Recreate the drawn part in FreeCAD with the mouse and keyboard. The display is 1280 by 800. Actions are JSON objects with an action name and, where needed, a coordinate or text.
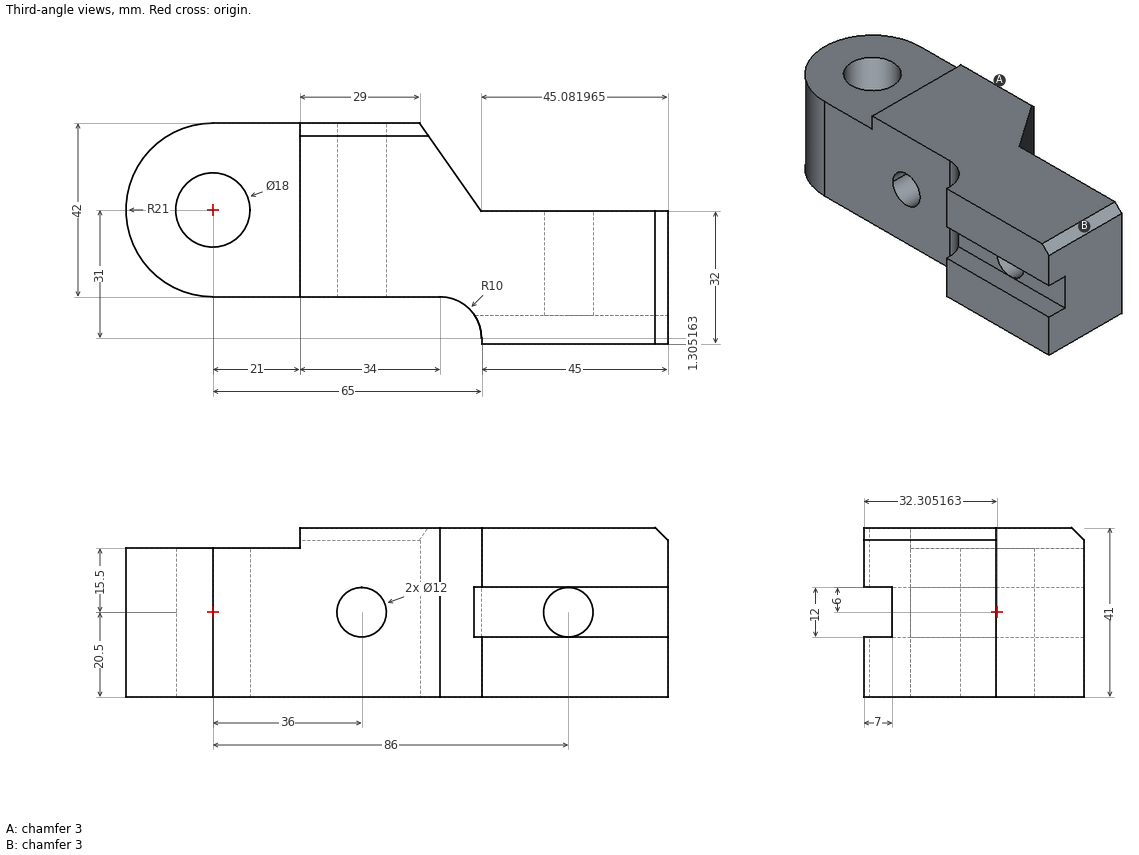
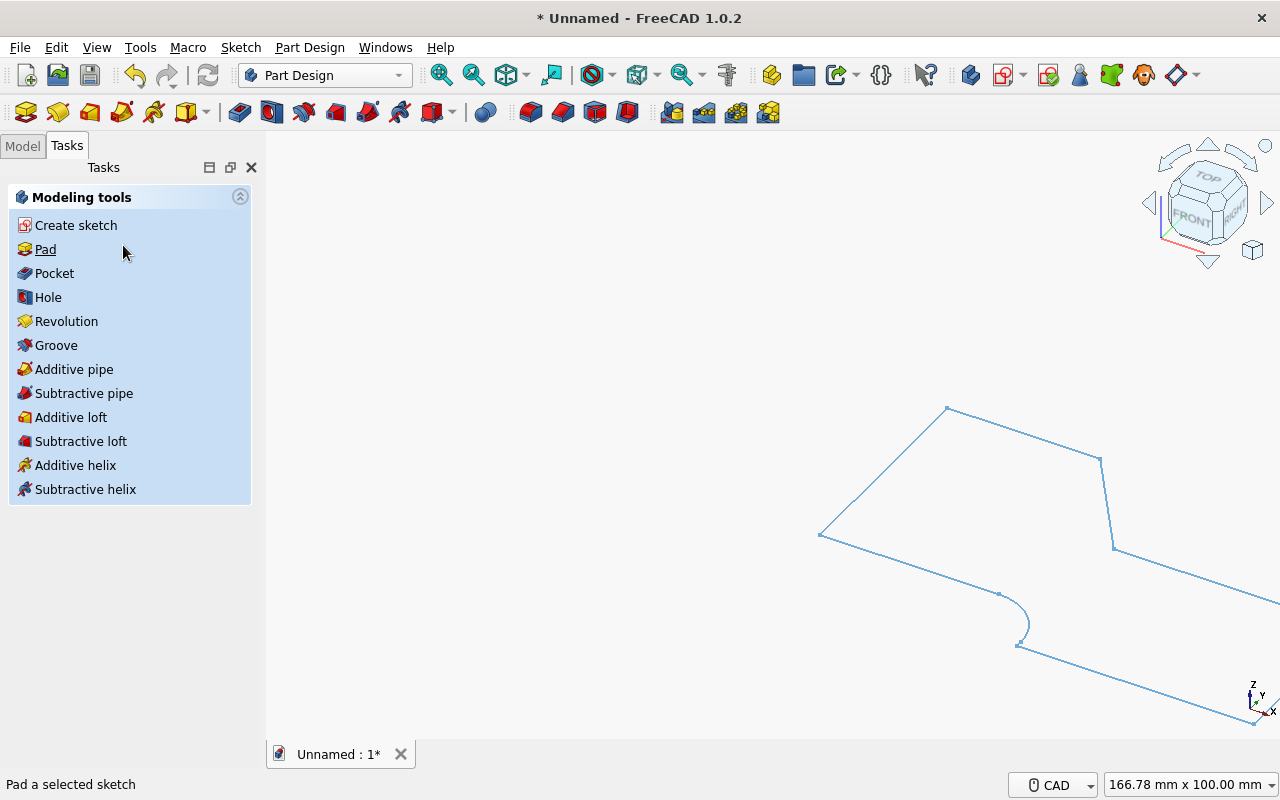
{"action": "left_click", "coordinate": [26, 112]}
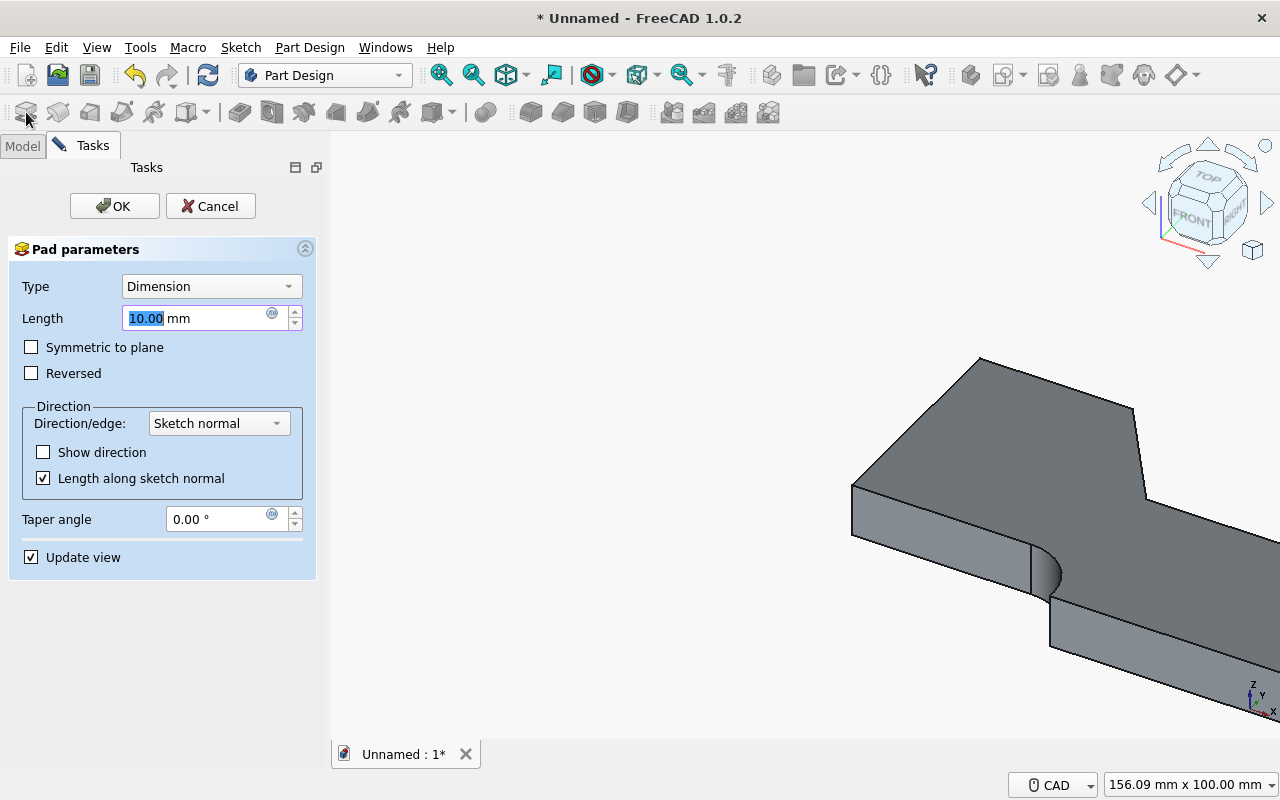
{"action": "type", "text": "41"}
{"action": "key", "text": "Tab"}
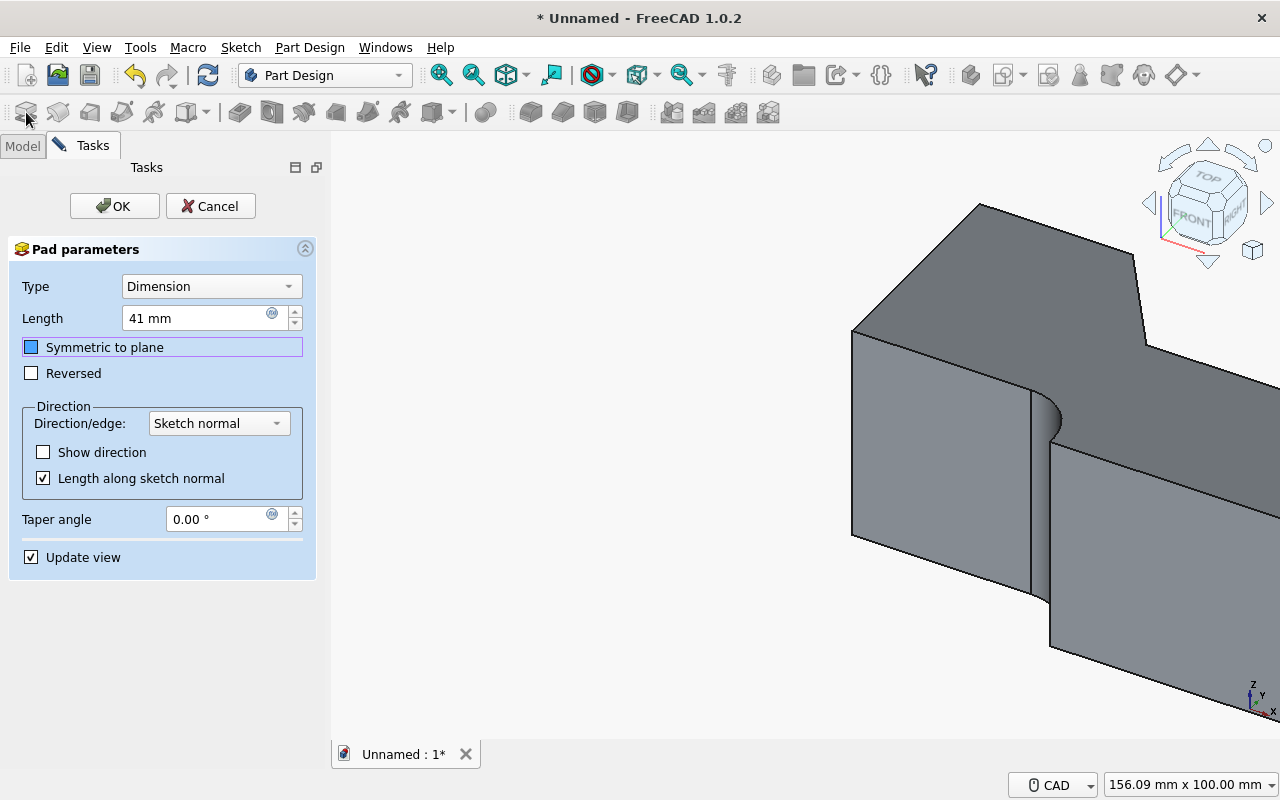
{"action": "left_click", "coordinate": [30, 347]}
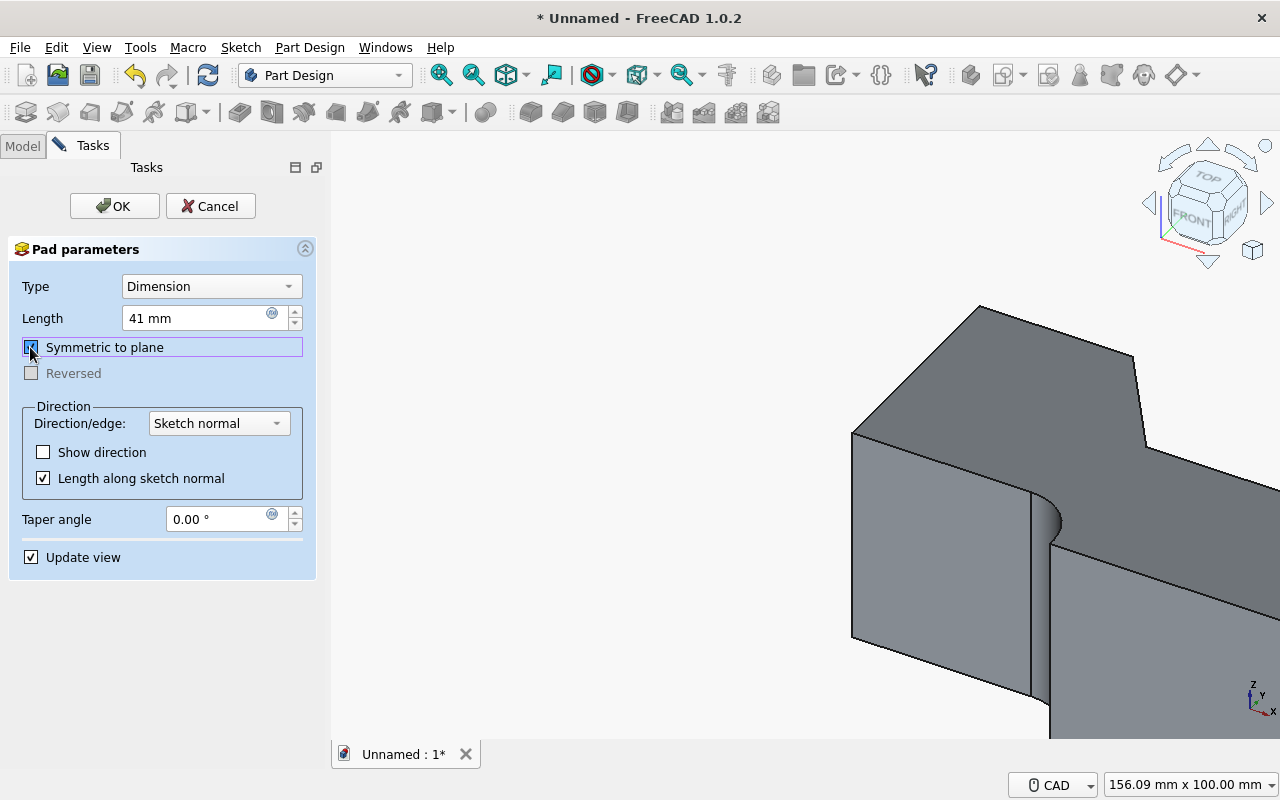
{"action": "left_click", "coordinate": [115, 206]}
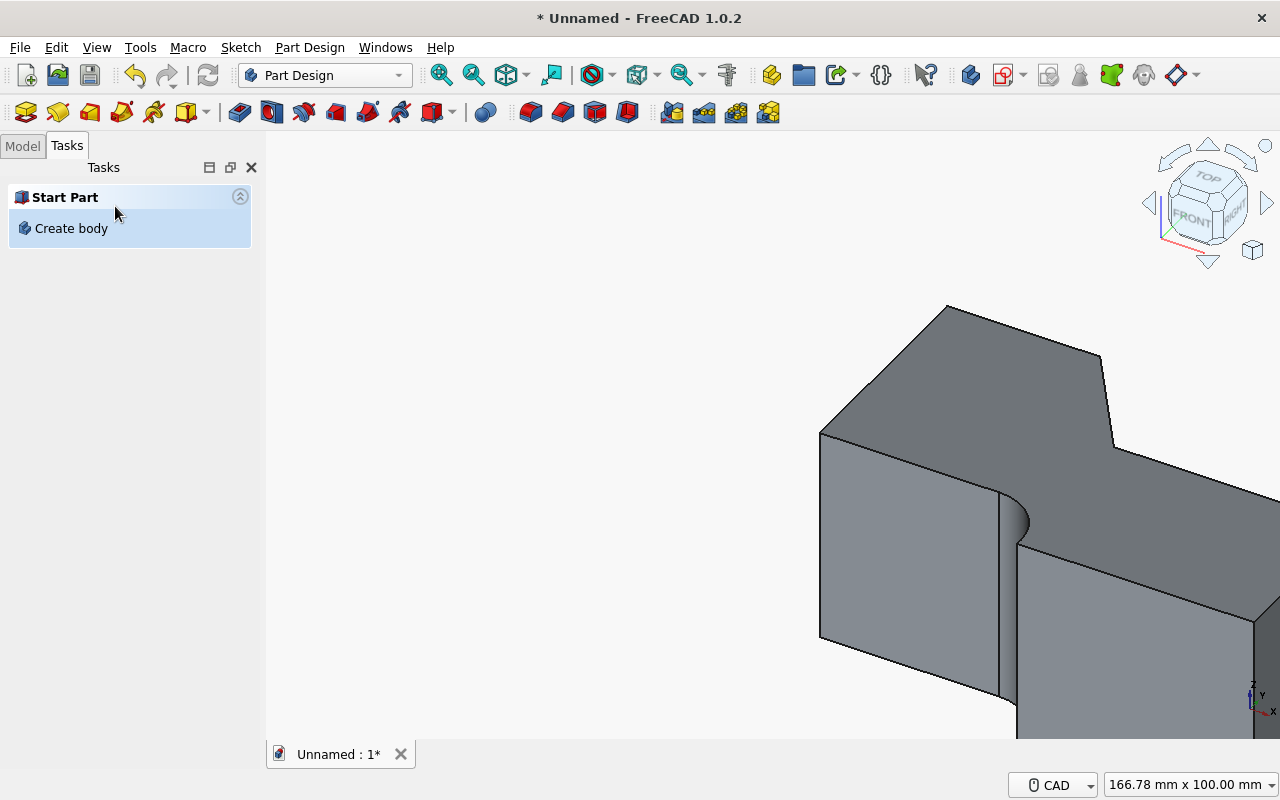
{"action": "left_click", "coordinate": [442, 76]}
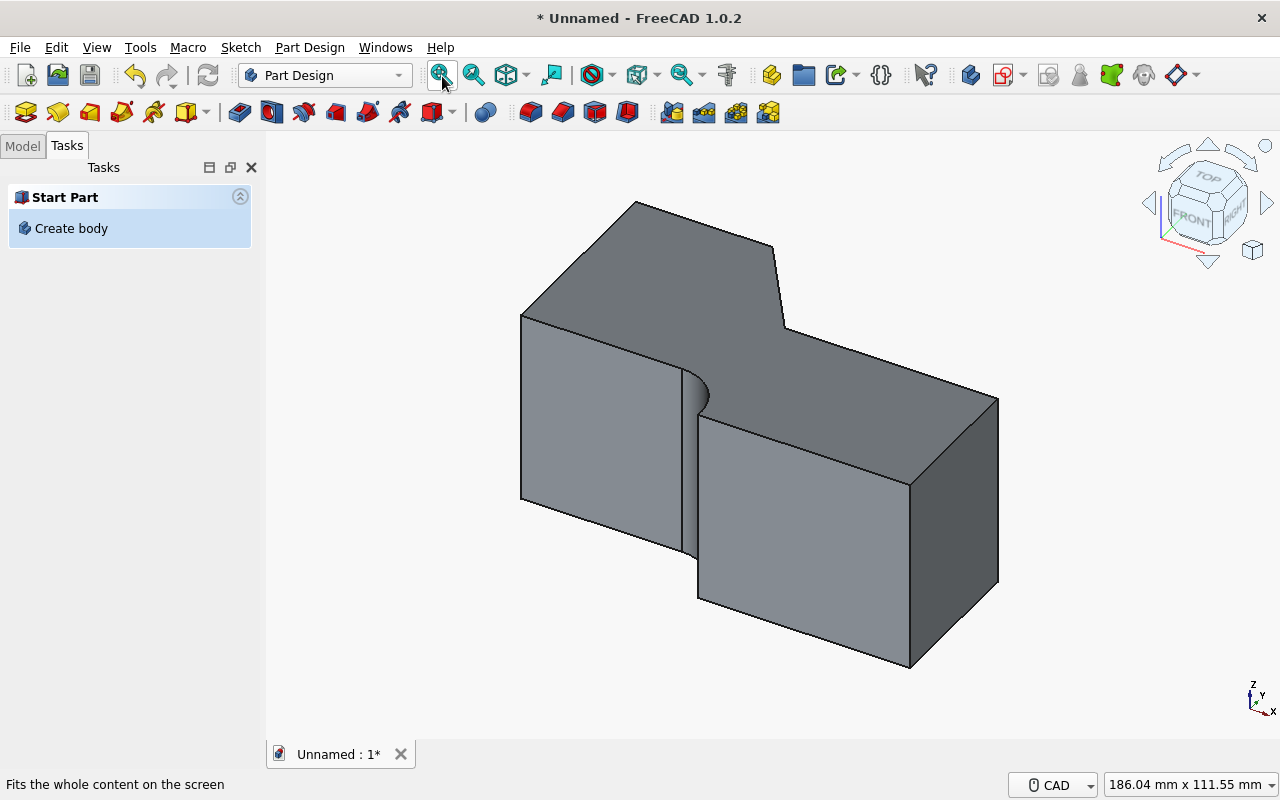
{"action": "left_click", "coordinate": [1004, 76]}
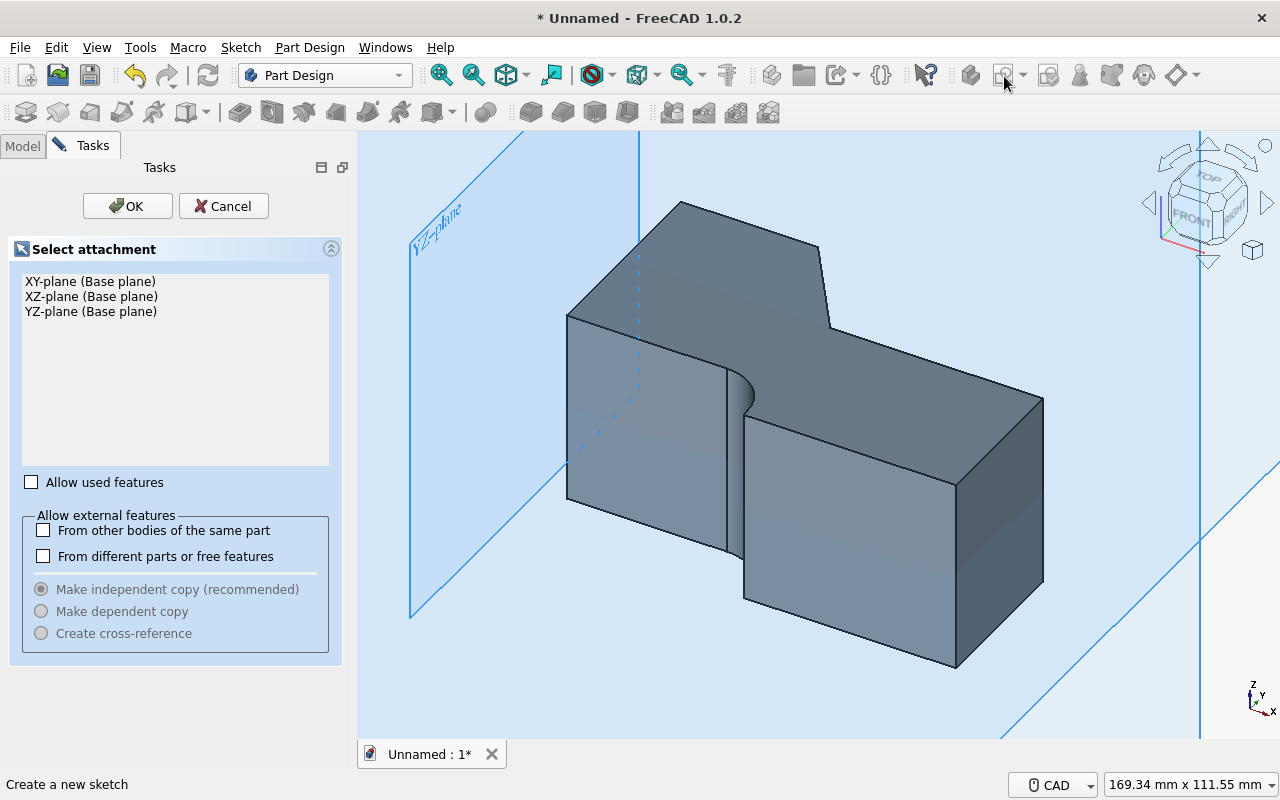
{"action": "left_click", "coordinate": [82, 282]}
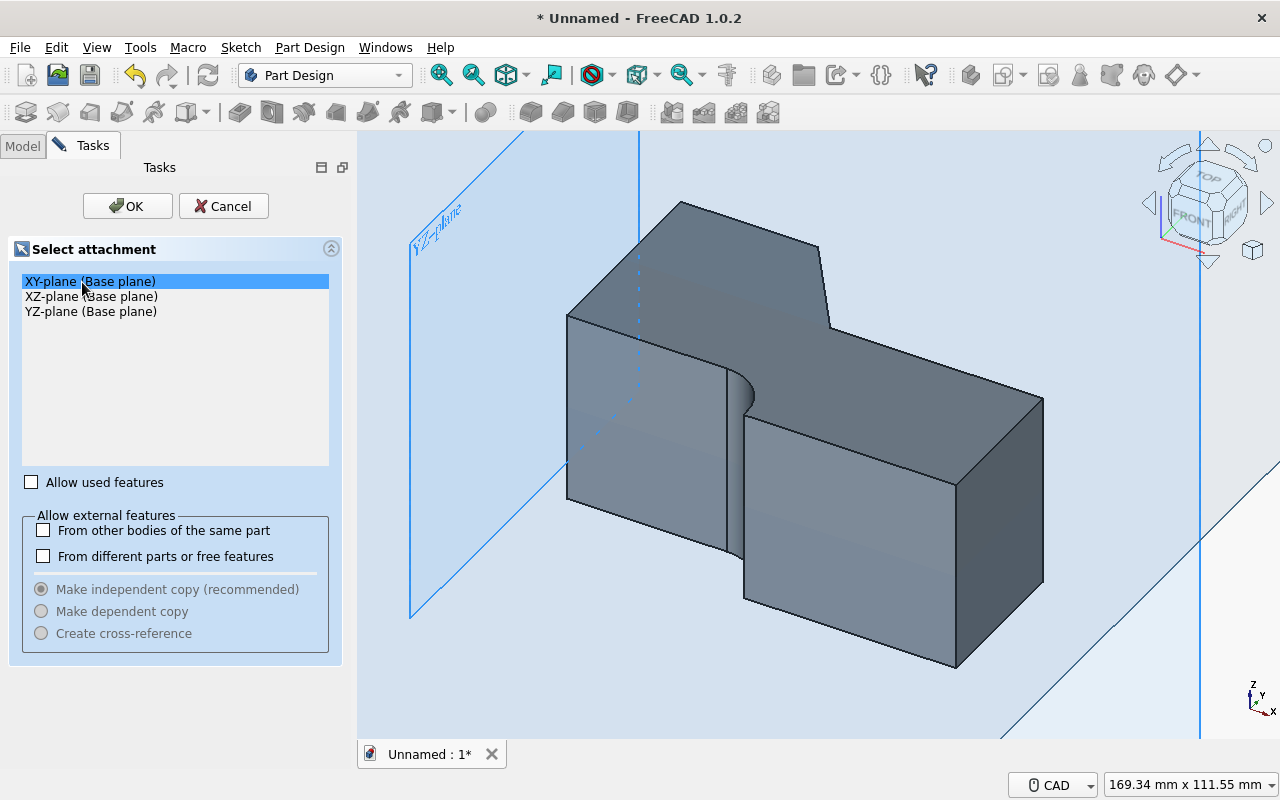
{"action": "left_click", "coordinate": [128, 206]}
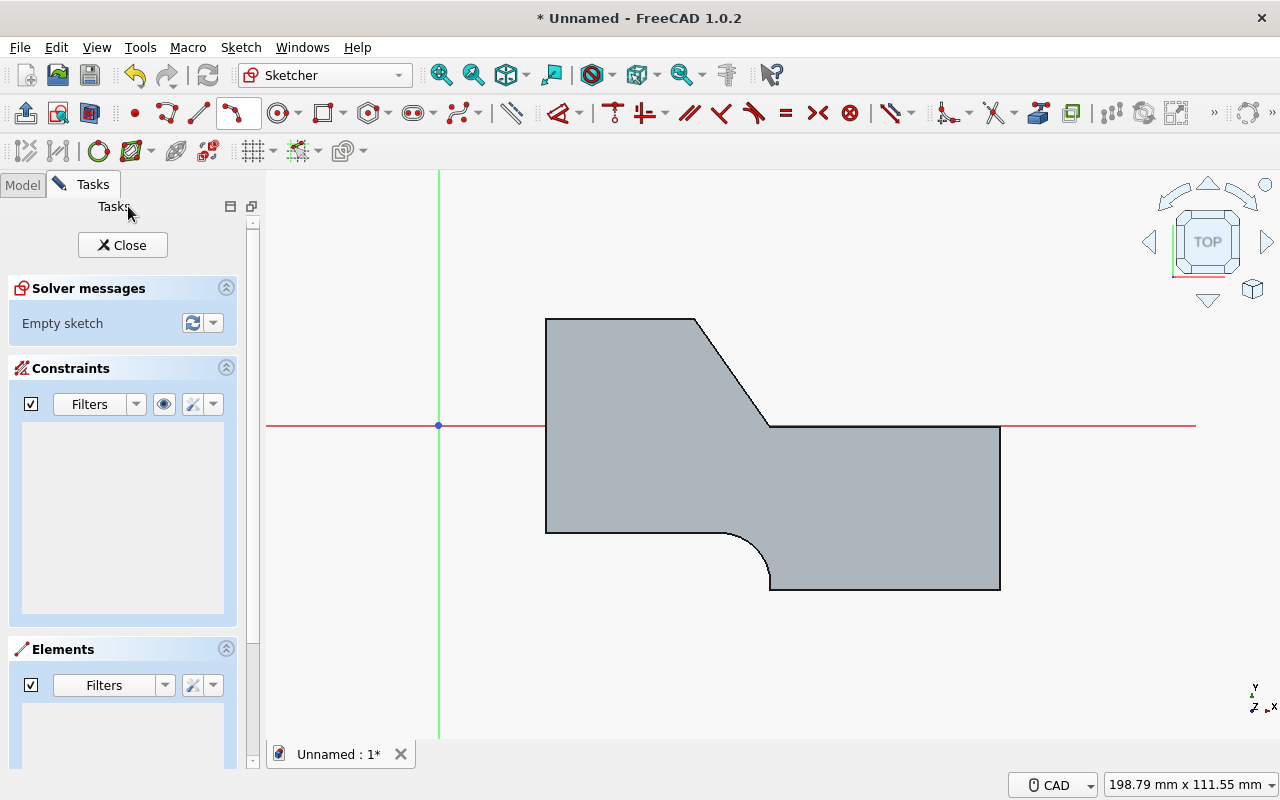
{"action": "left_click", "coordinate": [90, 114]}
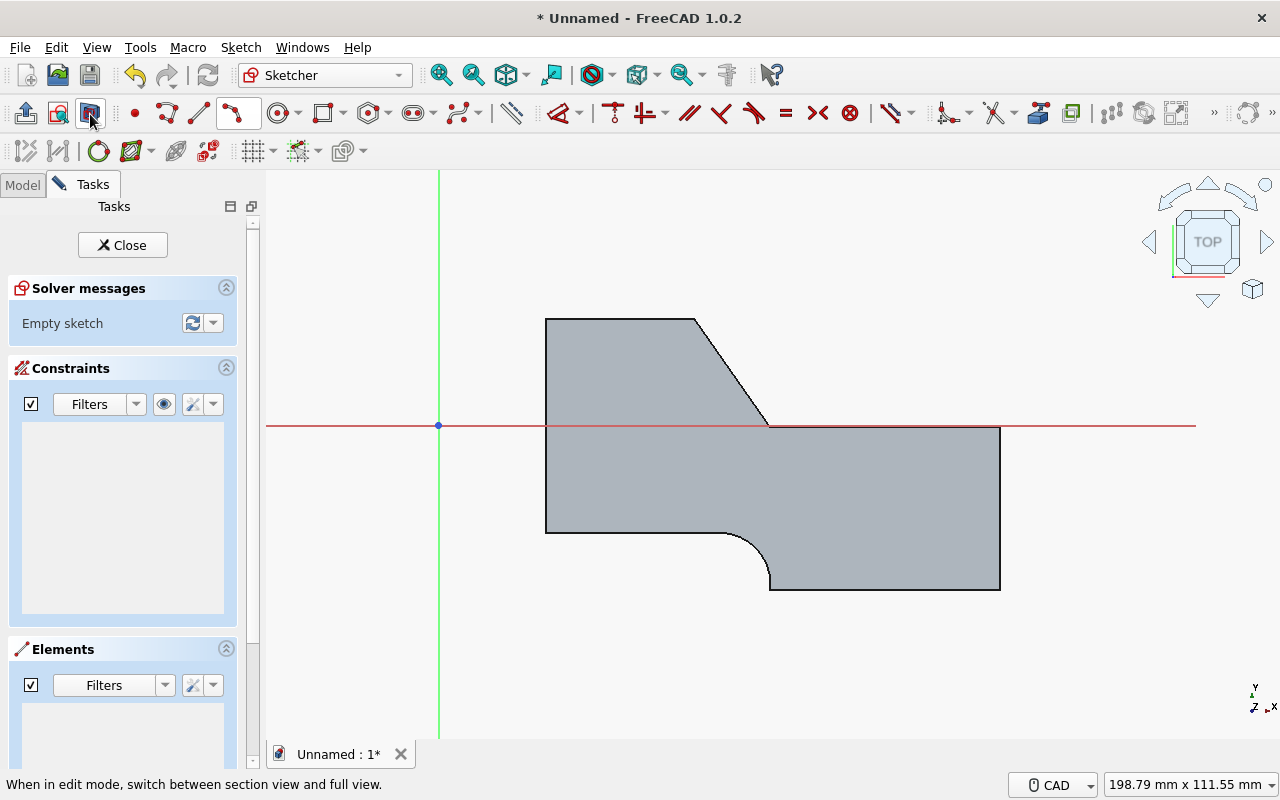
{"action": "scroll", "coordinate": [294, 391], "scroll_direction": "up", "scroll_amount": 3}